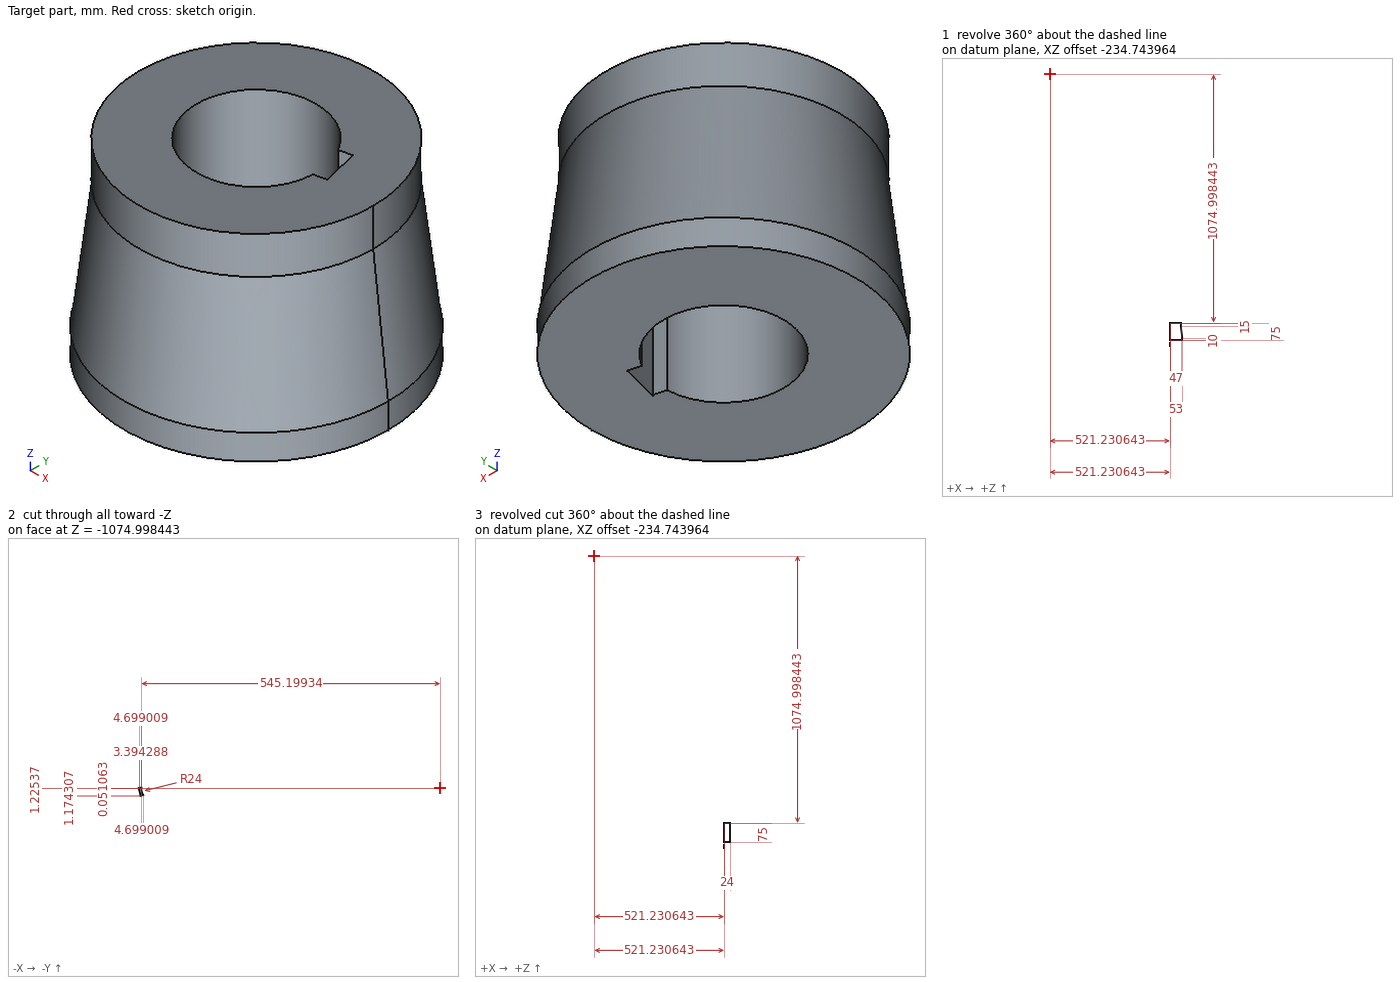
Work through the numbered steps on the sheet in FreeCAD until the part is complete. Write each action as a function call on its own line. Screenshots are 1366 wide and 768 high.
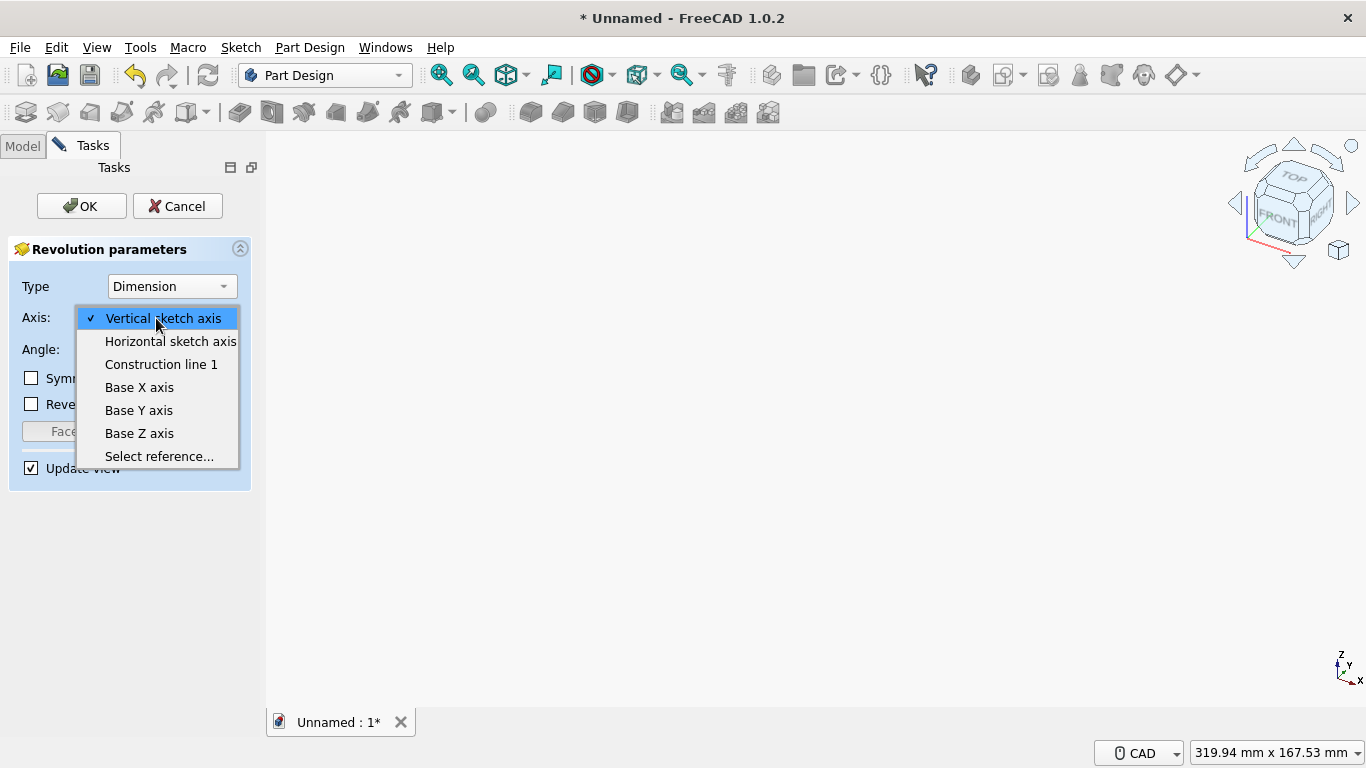
click(156, 364)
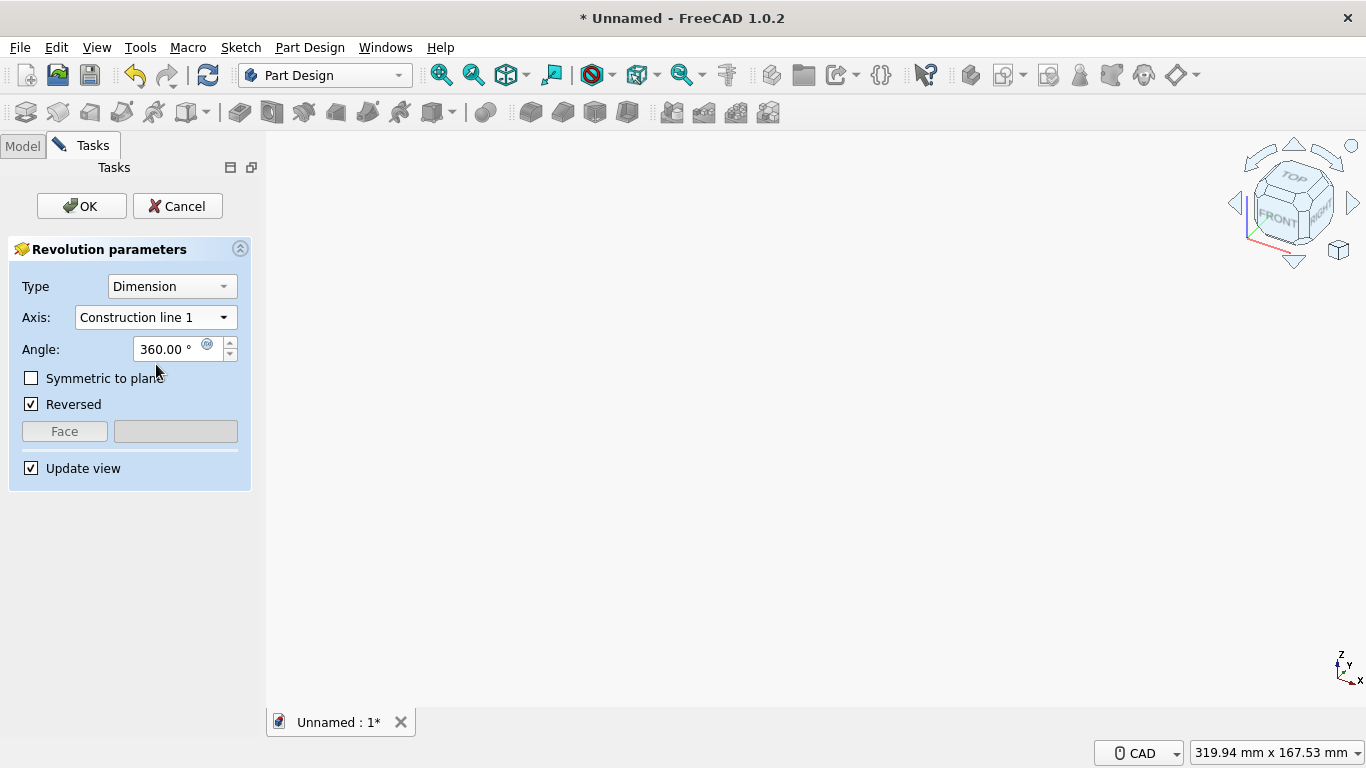
click(82, 206)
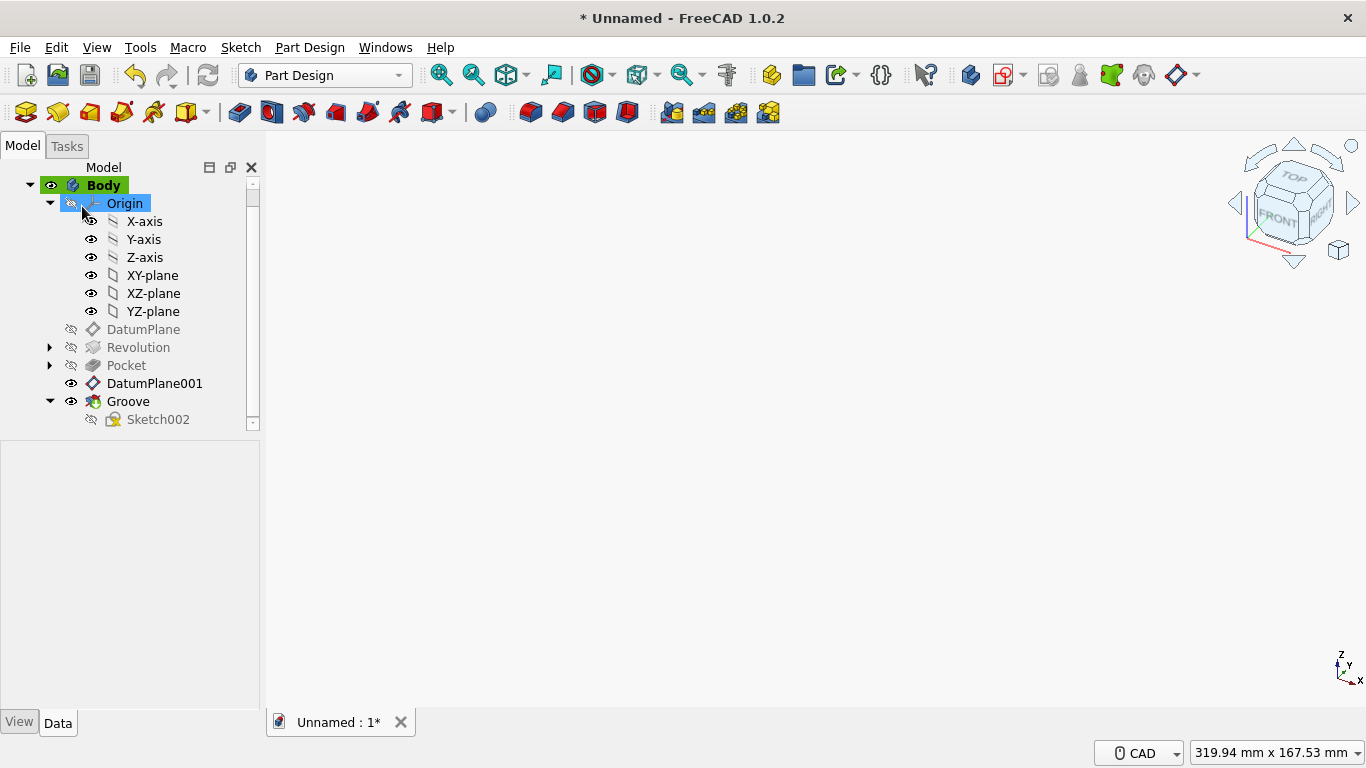
click(116, 383)
key(space)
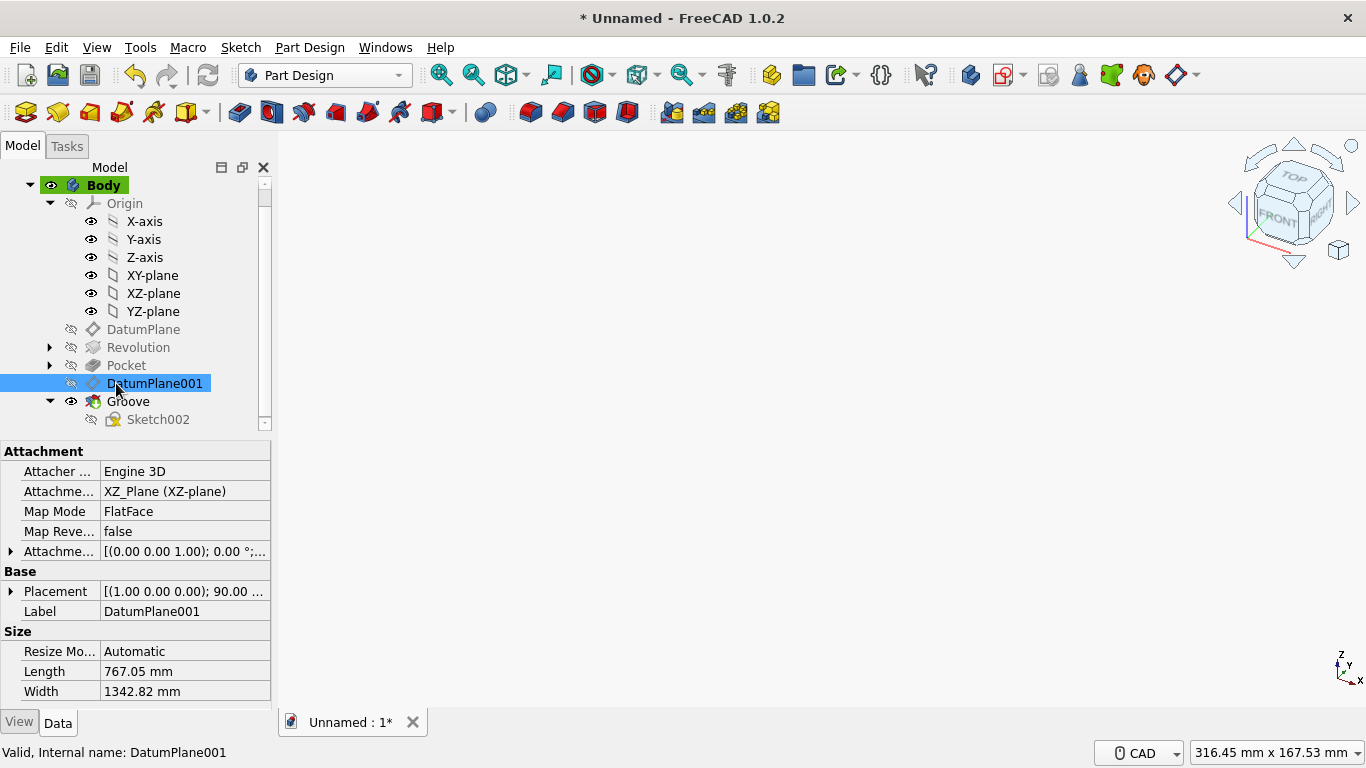
key(0)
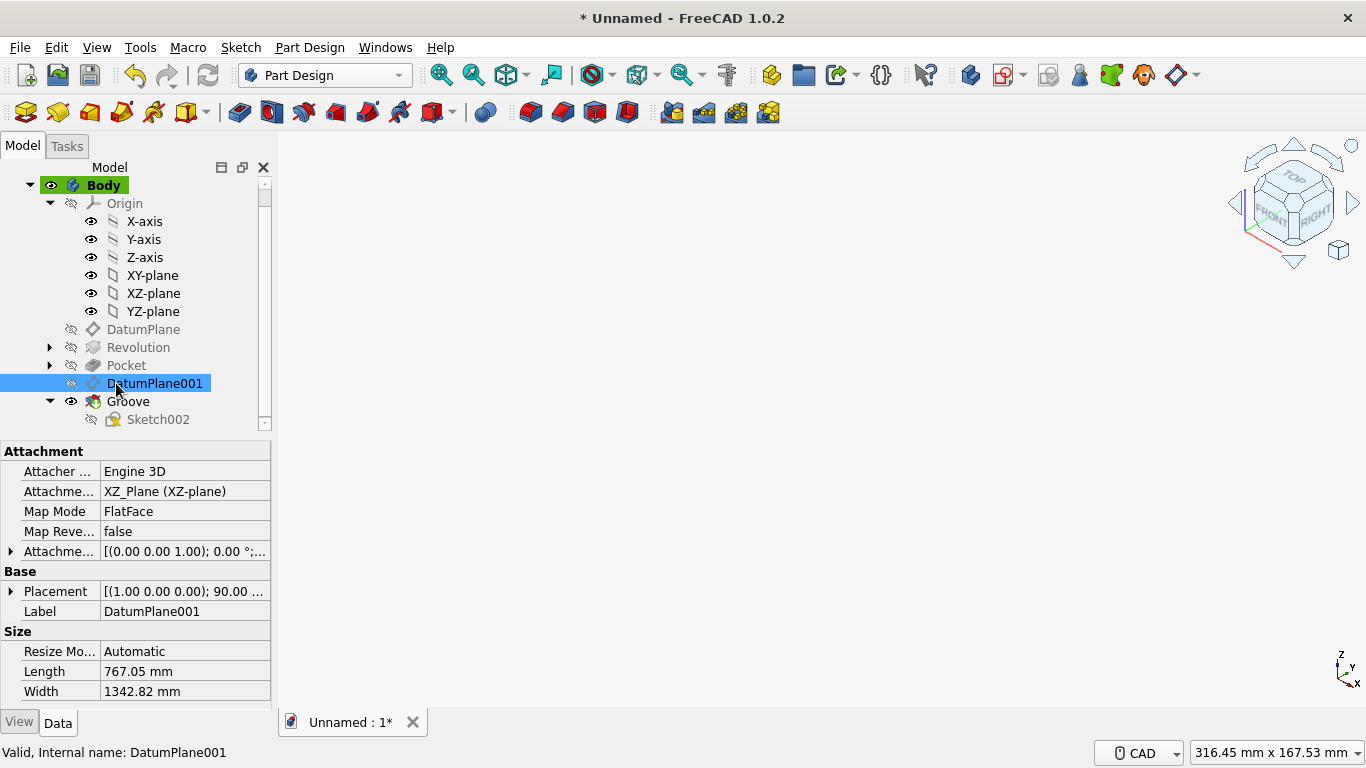
click(442, 76)